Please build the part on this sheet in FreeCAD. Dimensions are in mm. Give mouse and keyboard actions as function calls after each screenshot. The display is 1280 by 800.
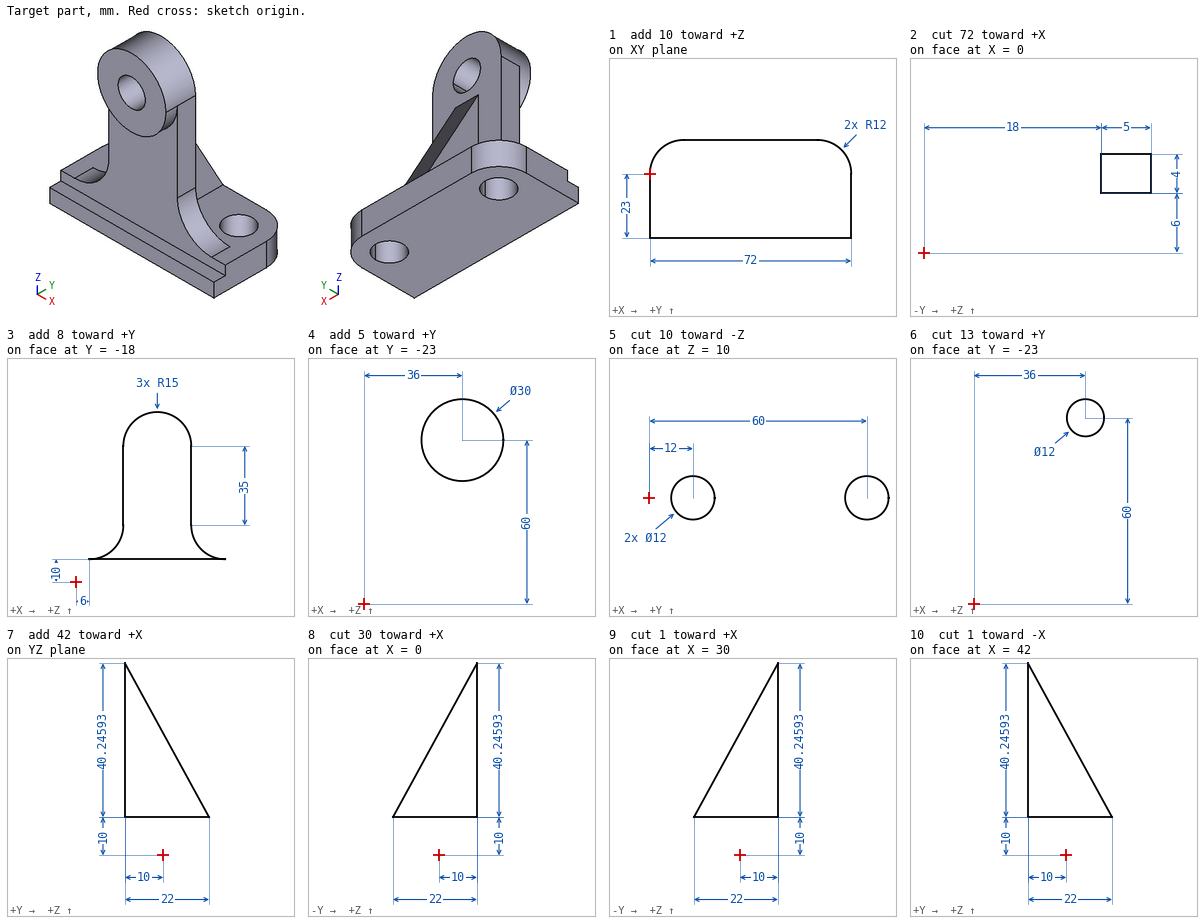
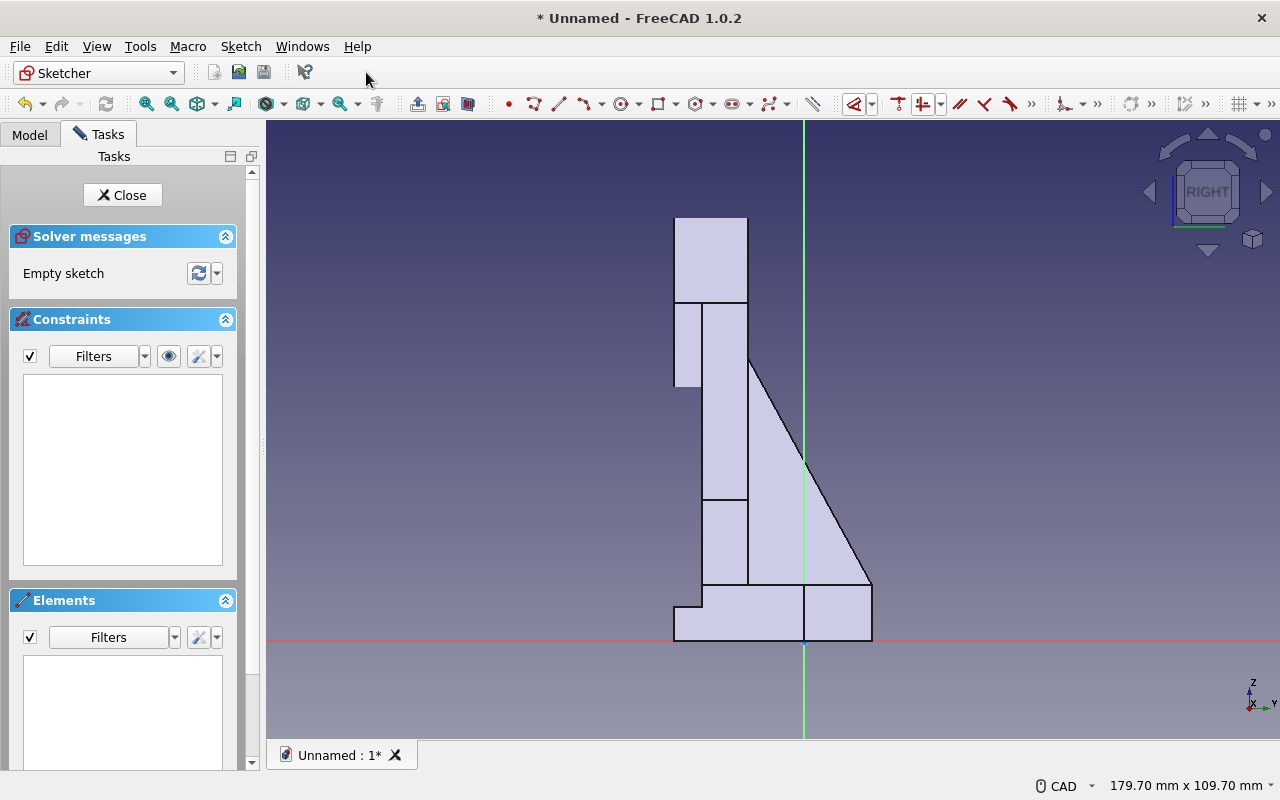
key(q)
key(s)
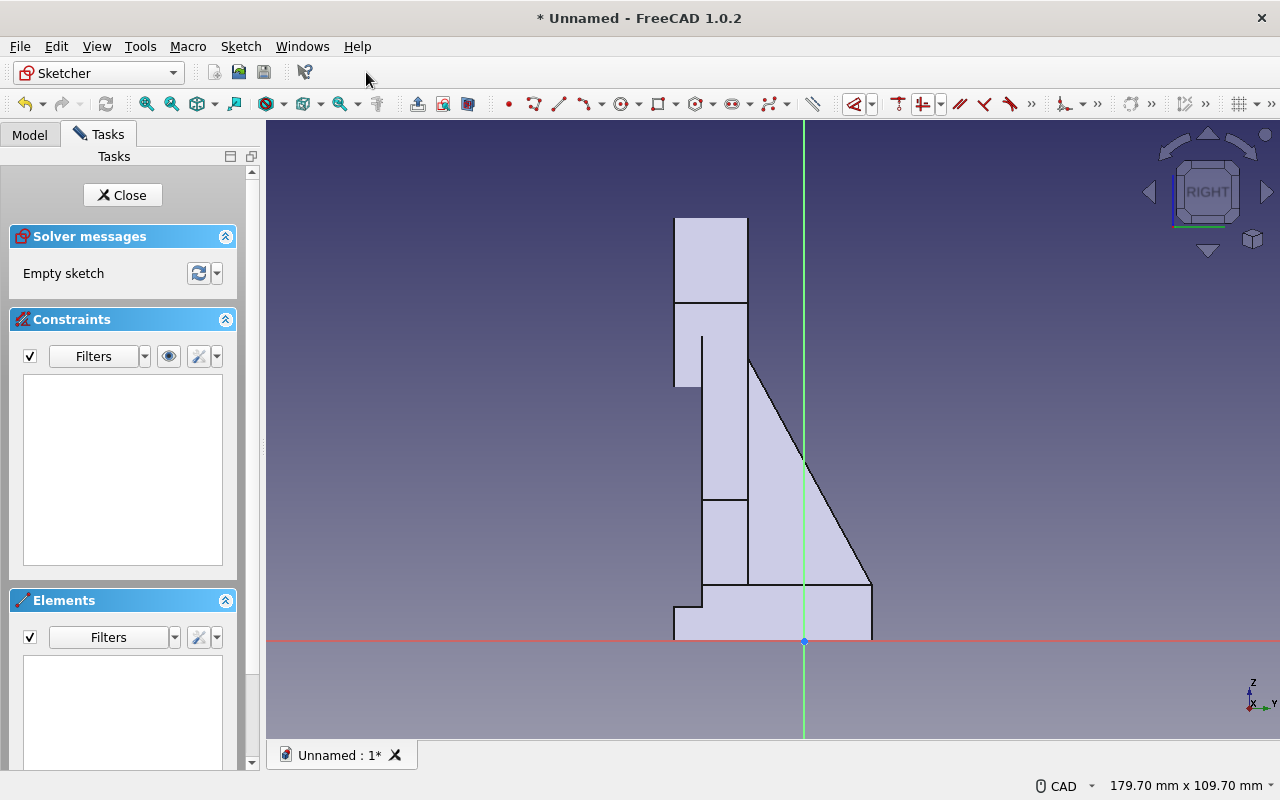
scroll(1024, 641, up, 2)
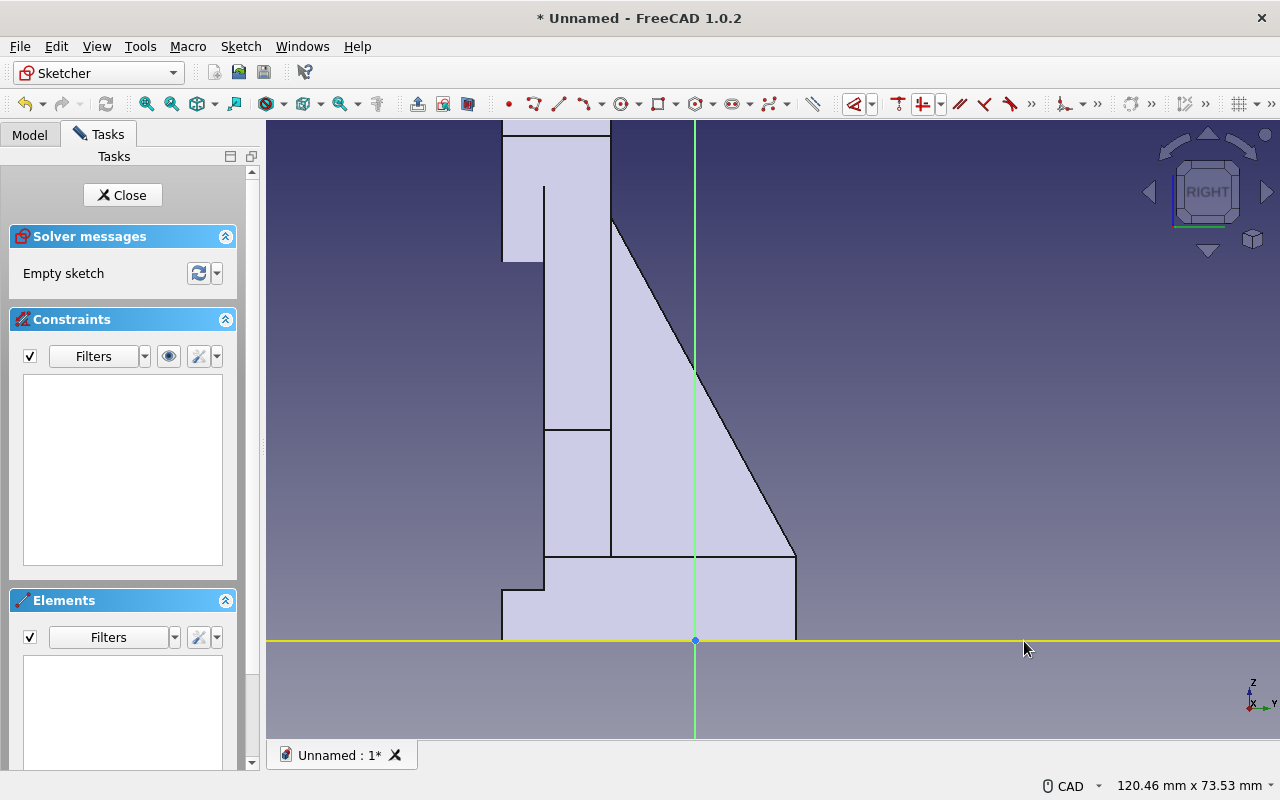
click(534, 104)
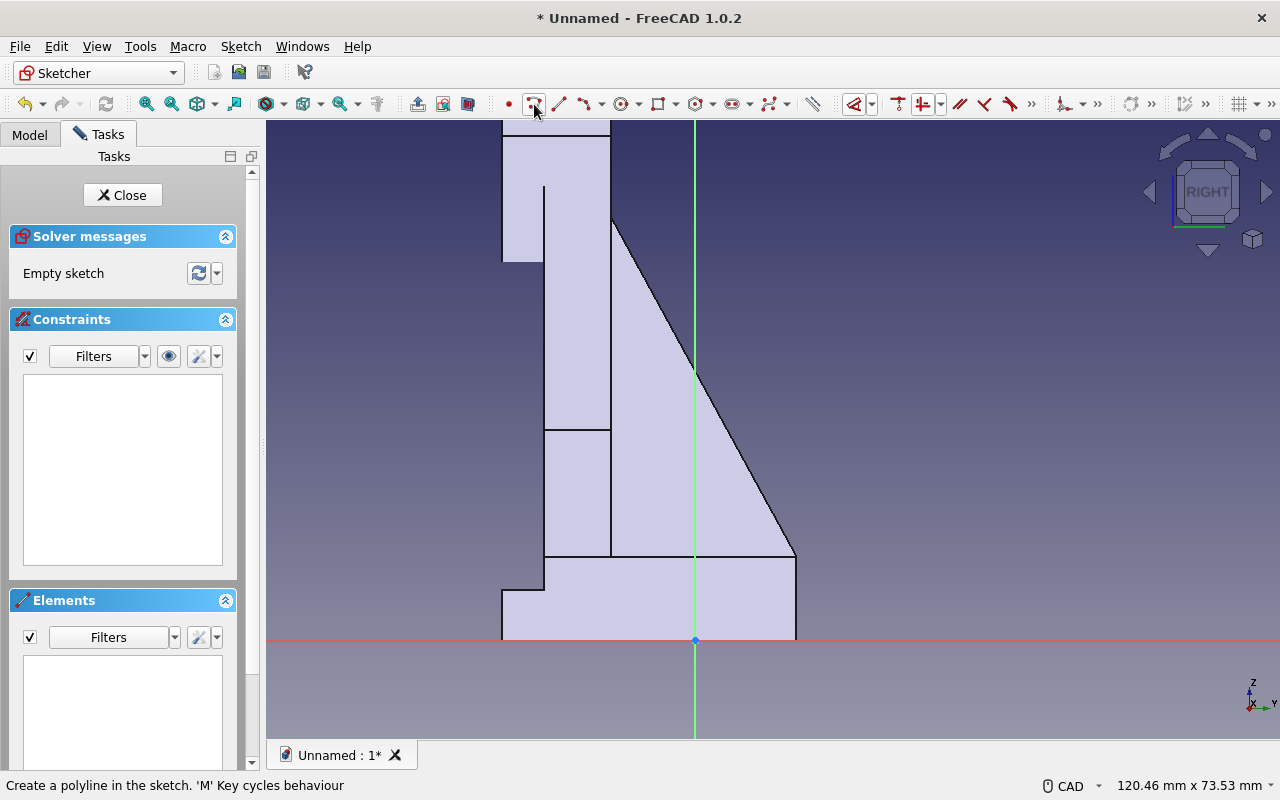
click(611, 557)
click(796, 557)
click(611, 218)
click(611, 558)
key(Escape)
key(Escape)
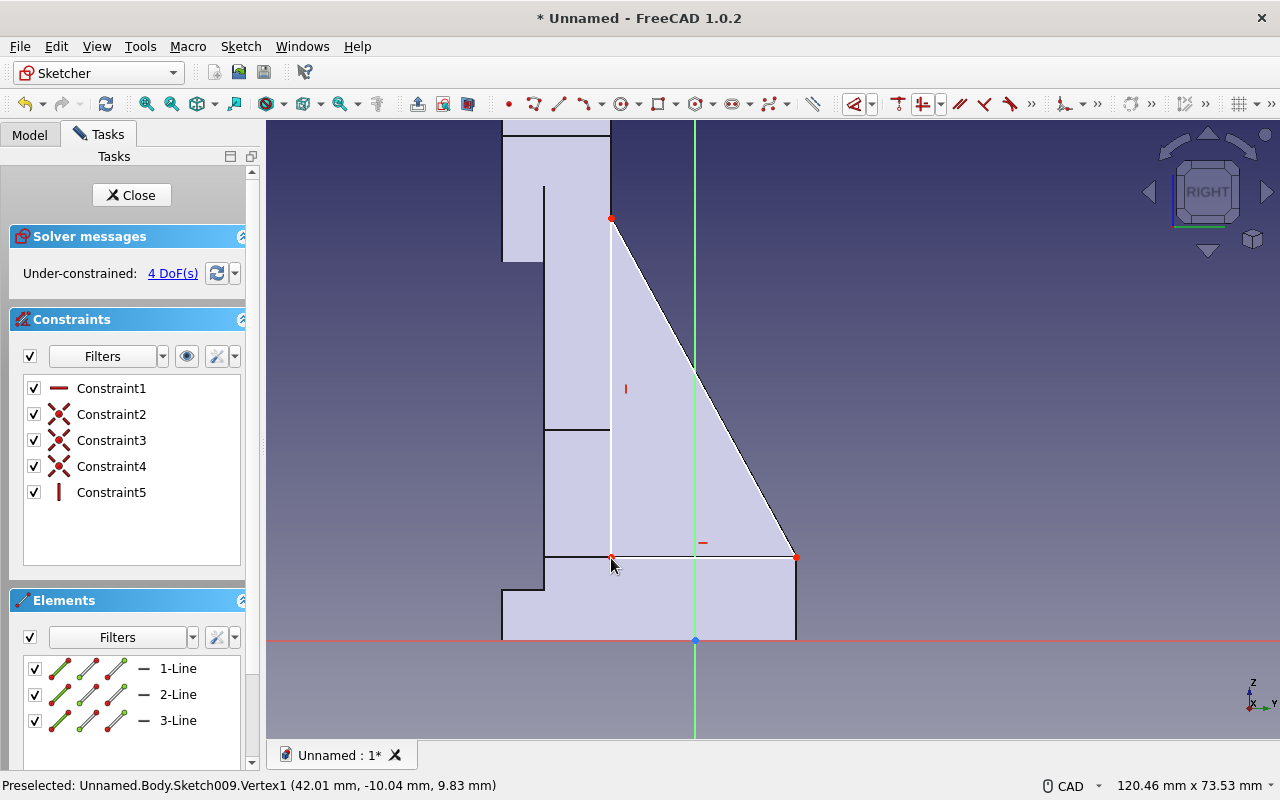
click(667, 558)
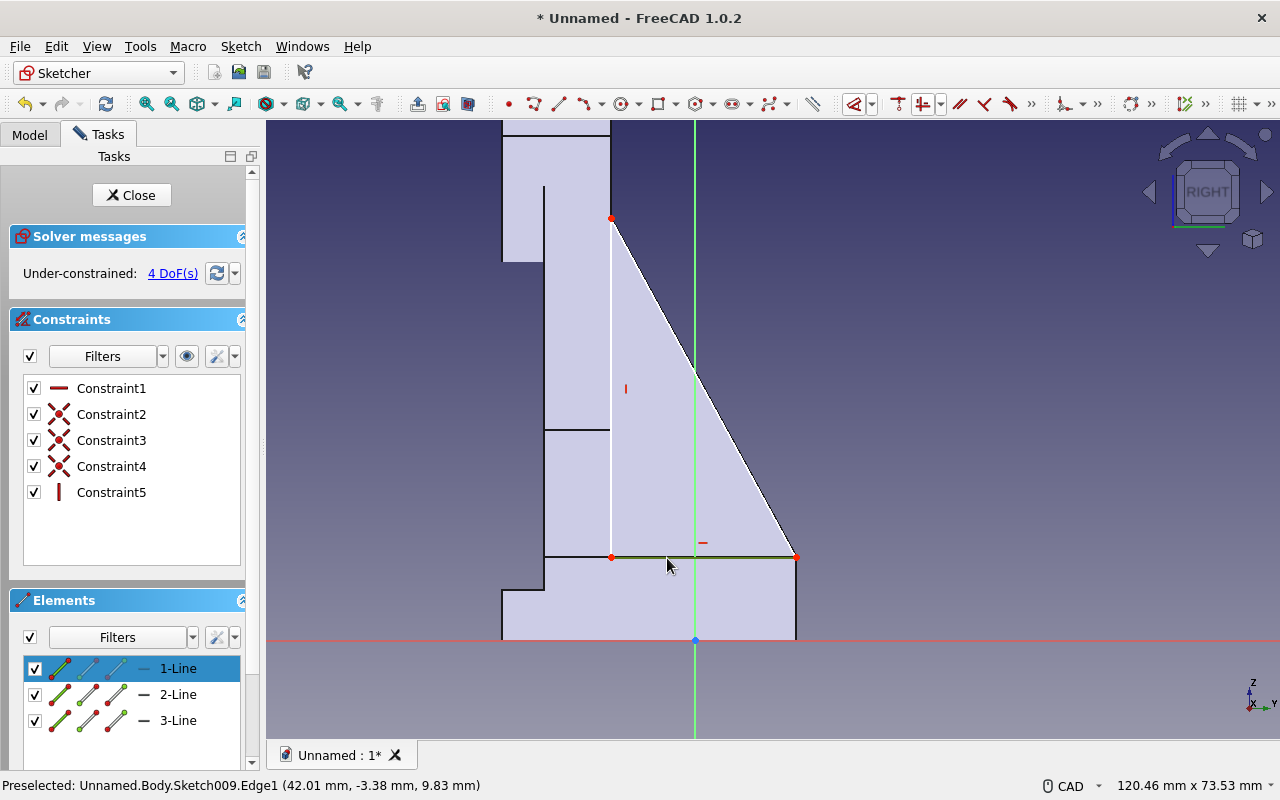
click(872, 104)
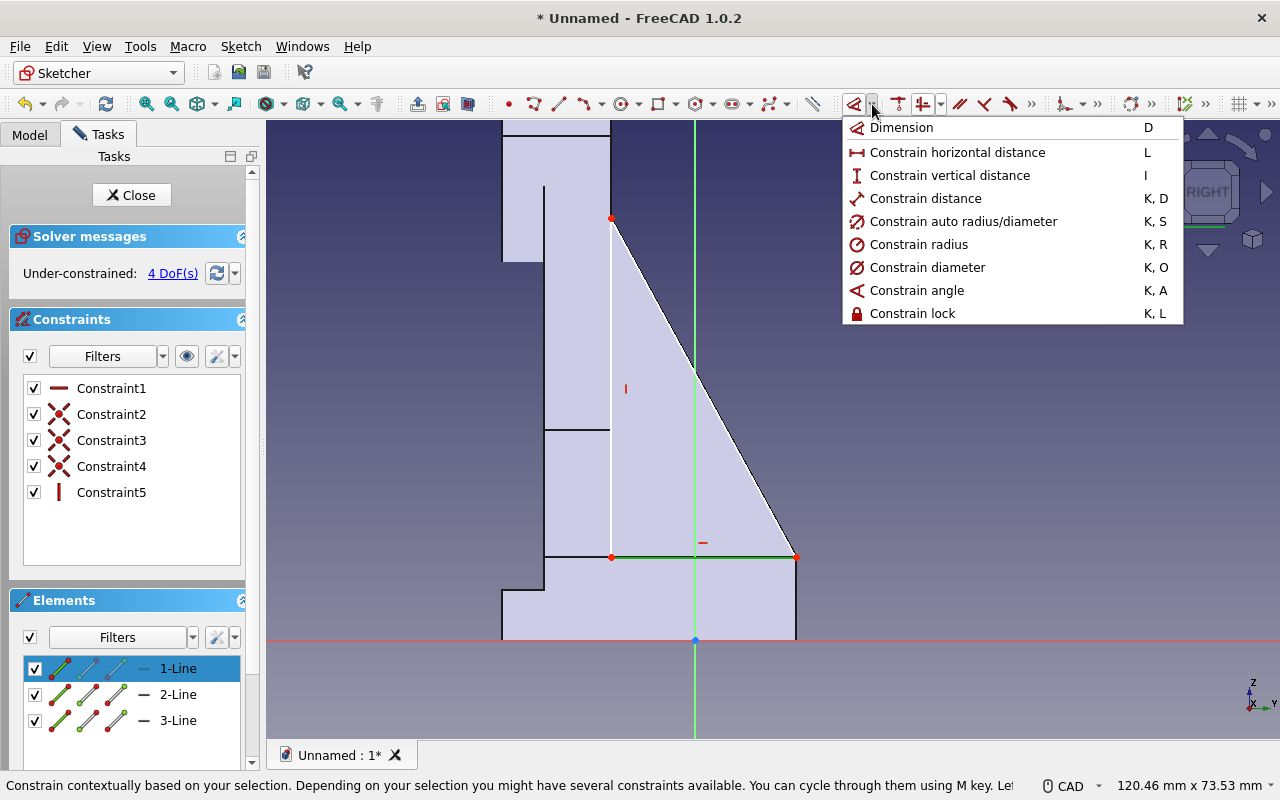
click(1013, 152)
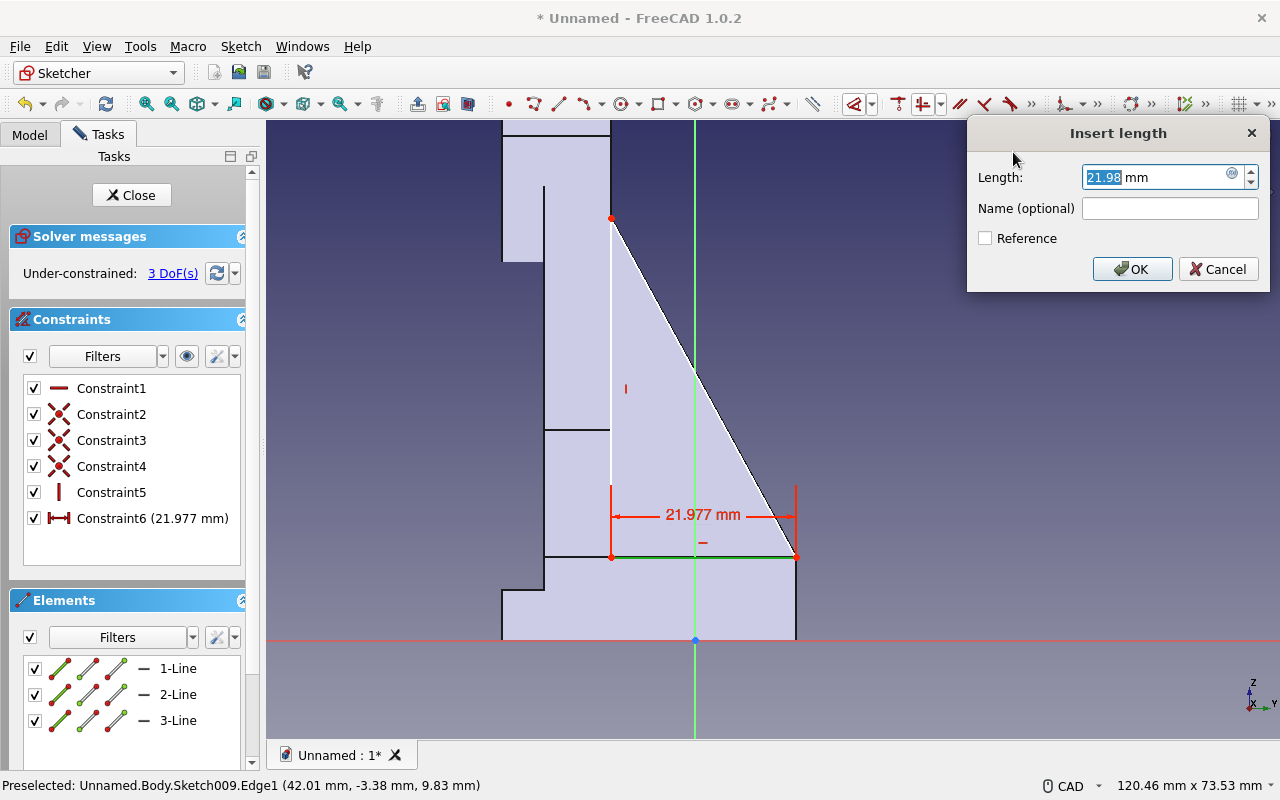
text(22)
key(Return)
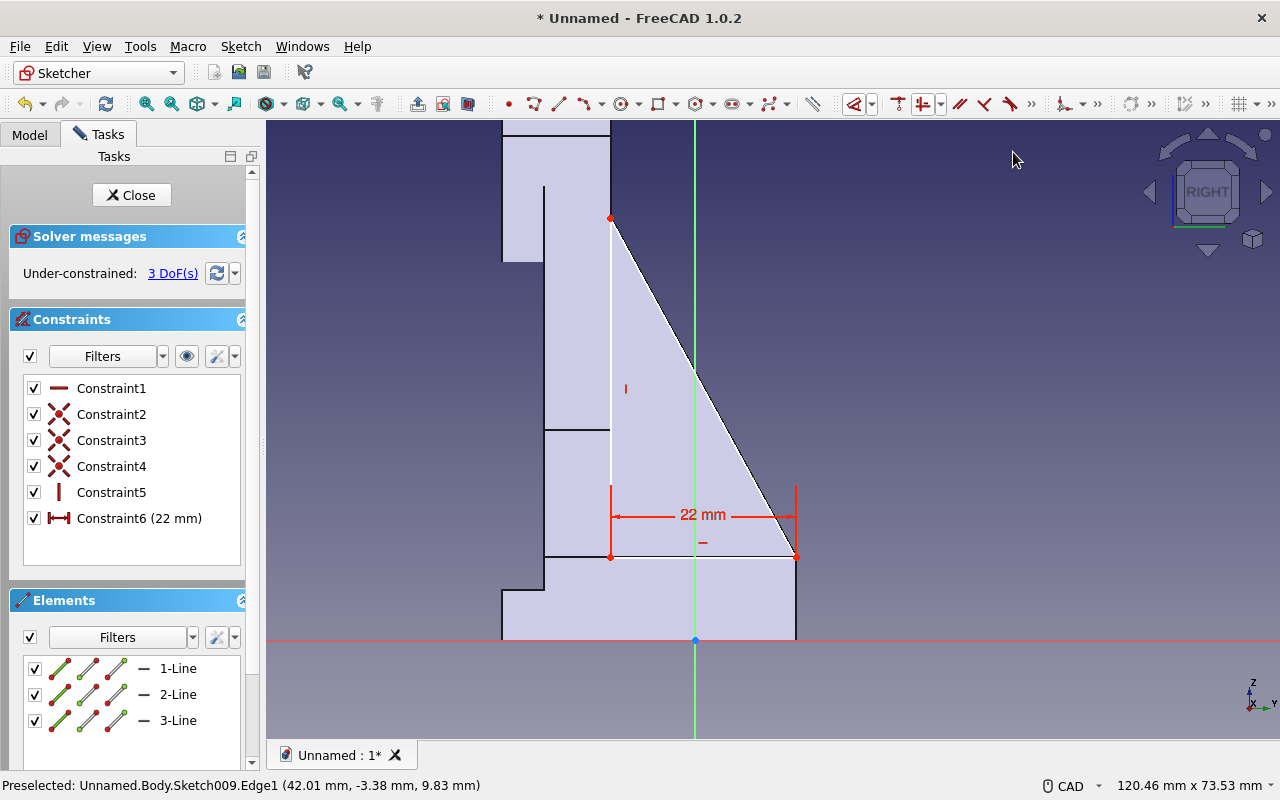
click(611, 558)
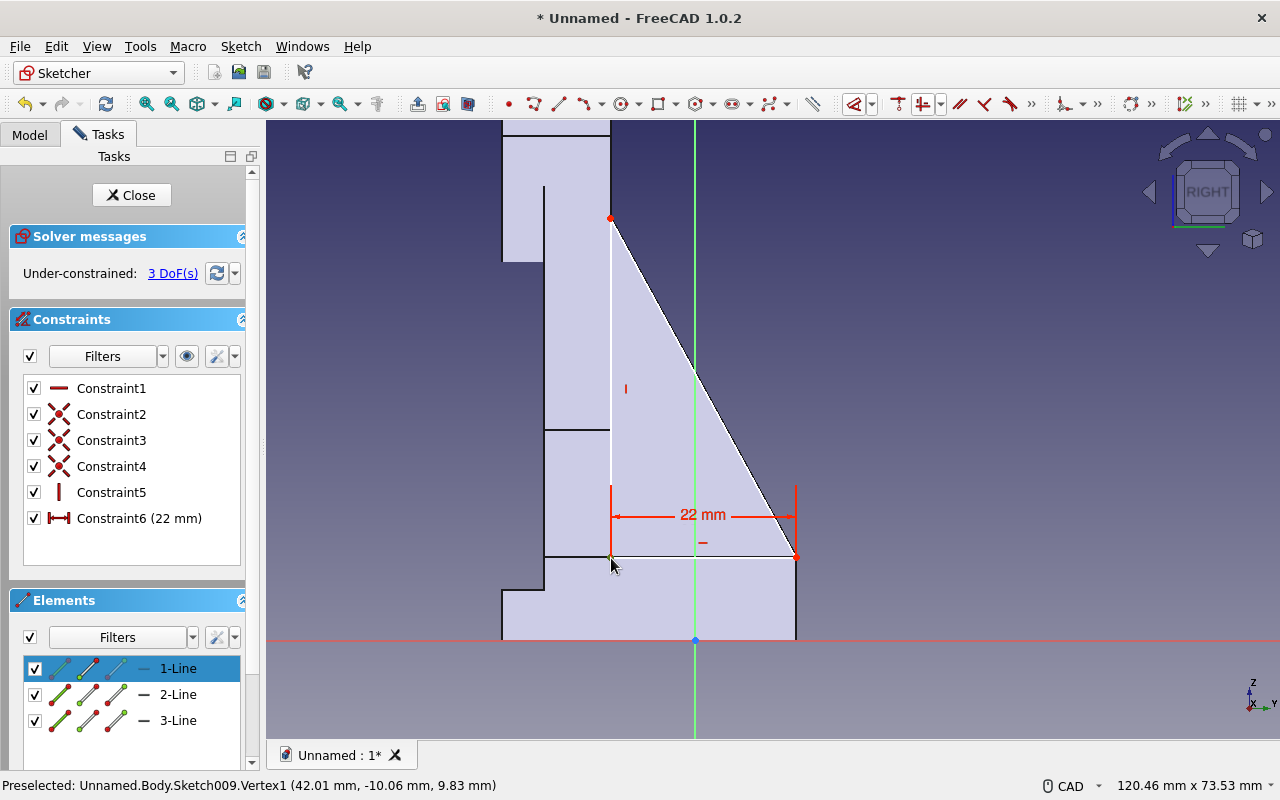
key(l)